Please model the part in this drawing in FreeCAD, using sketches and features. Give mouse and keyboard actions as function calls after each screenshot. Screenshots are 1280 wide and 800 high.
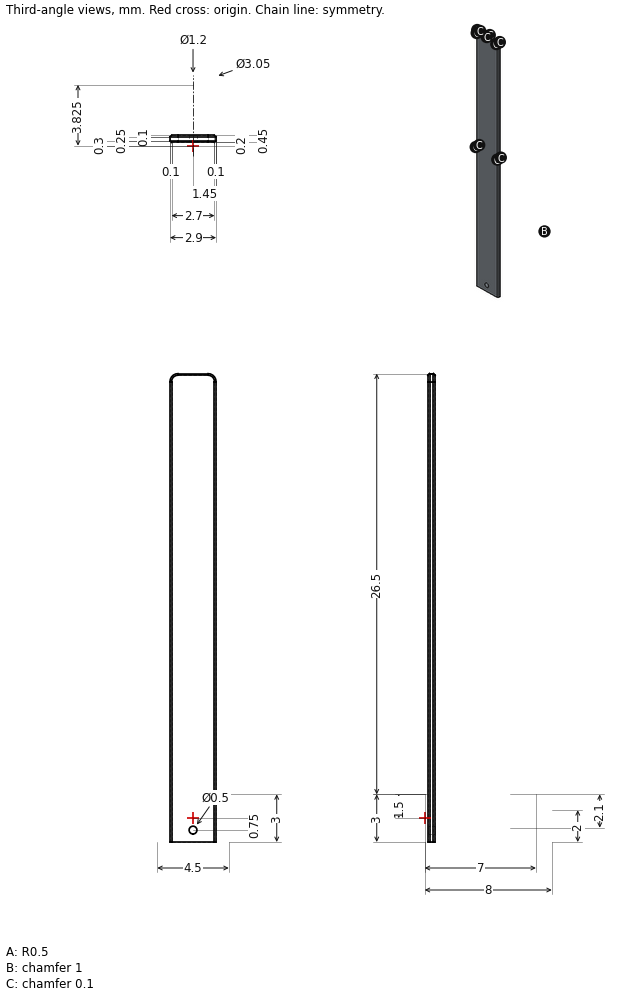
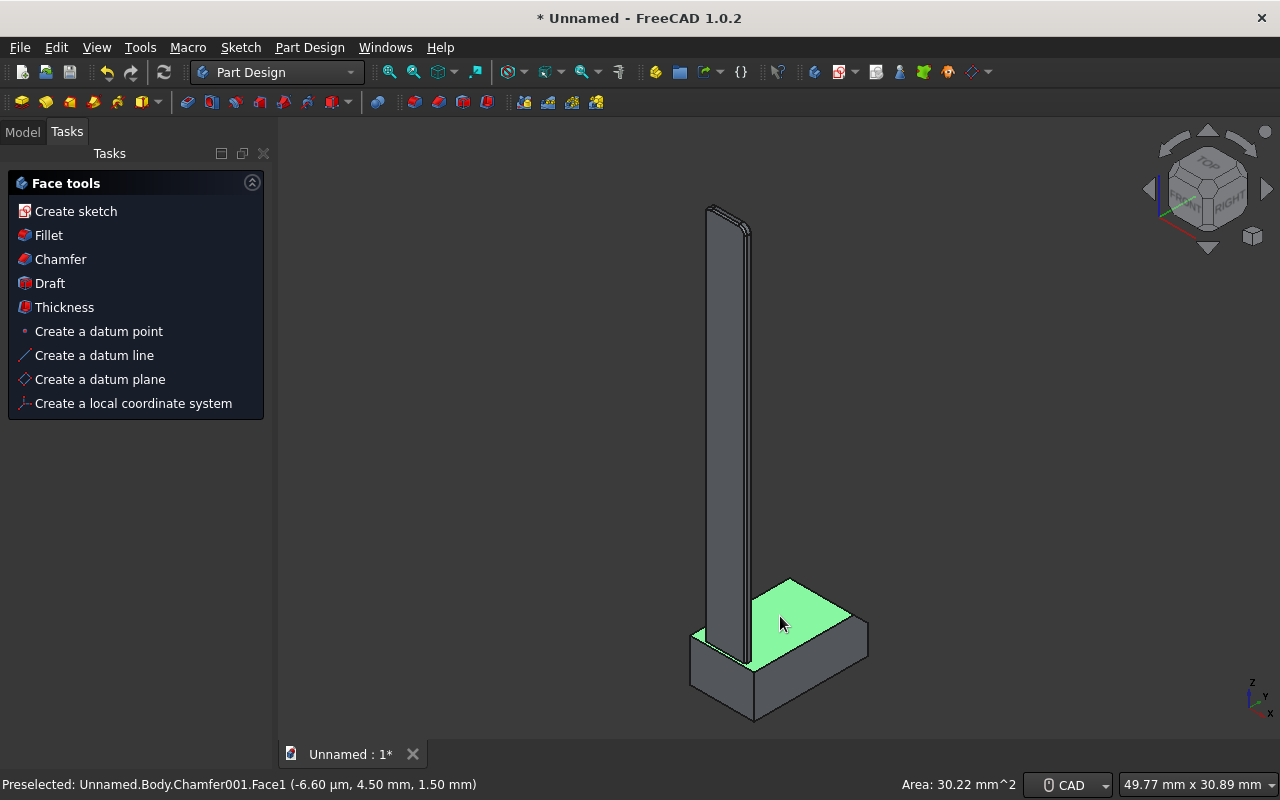
click(840, 72)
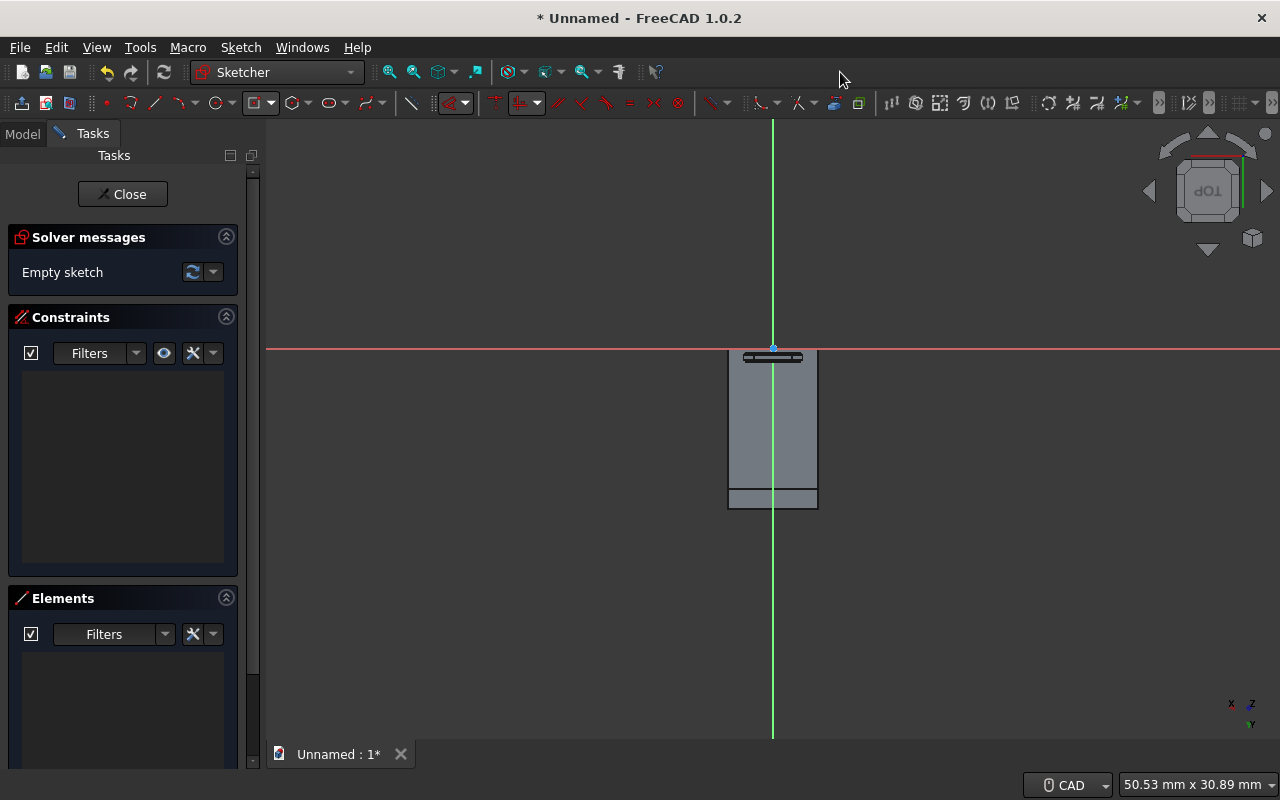
key(q)
key(s)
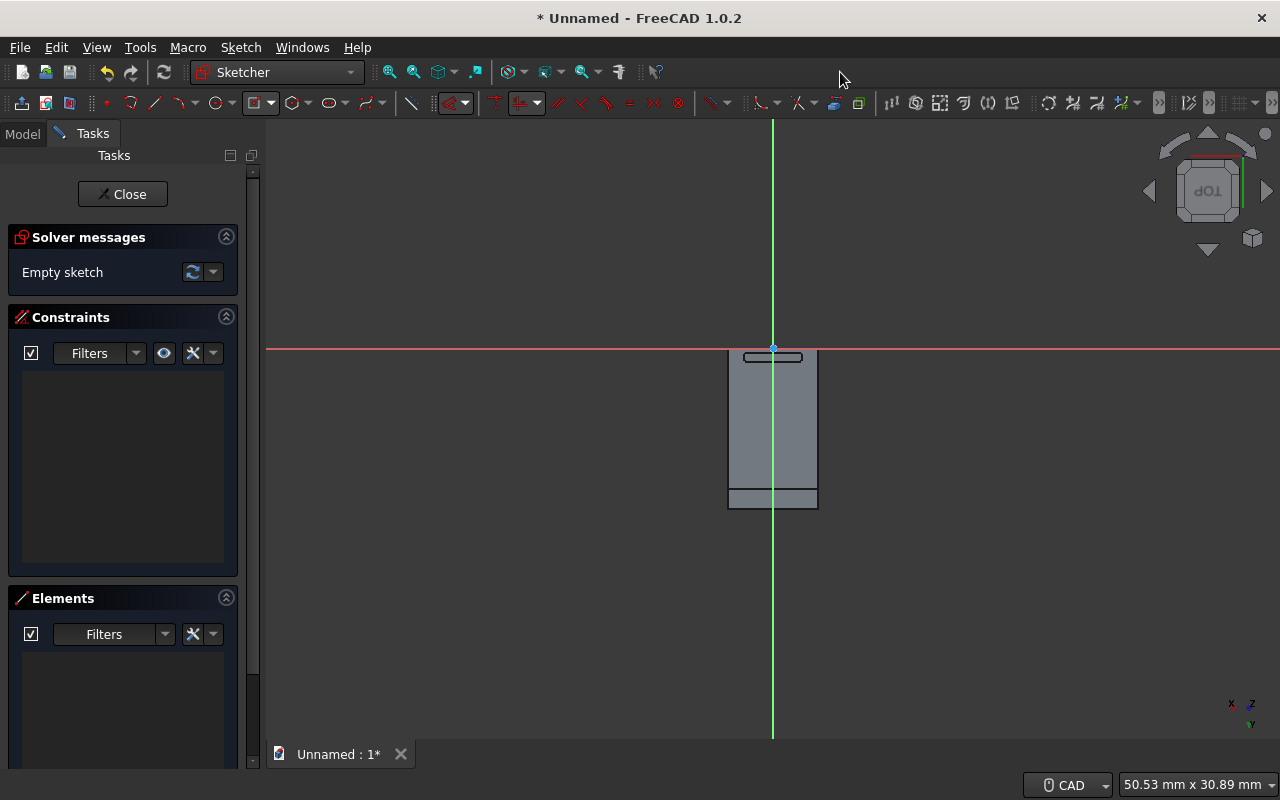
scroll(795, 394, up, 7)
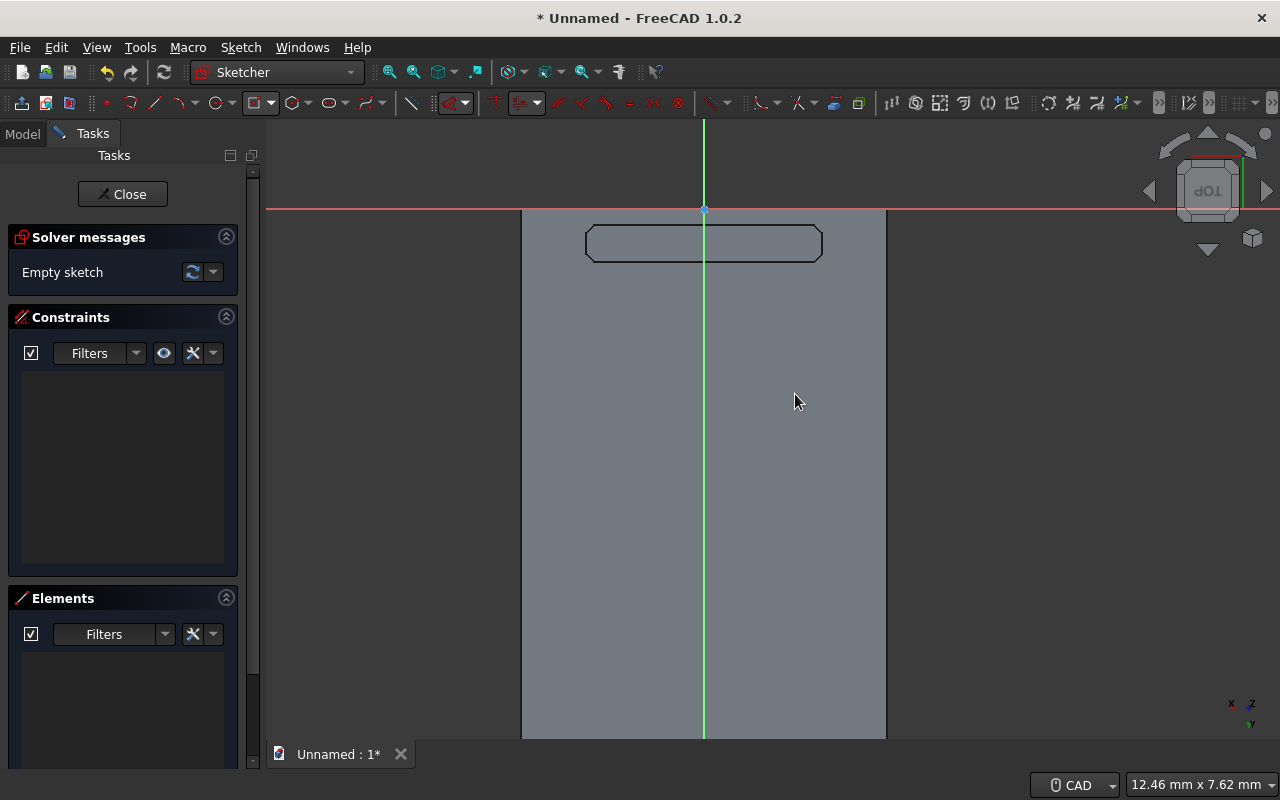
click(216, 104)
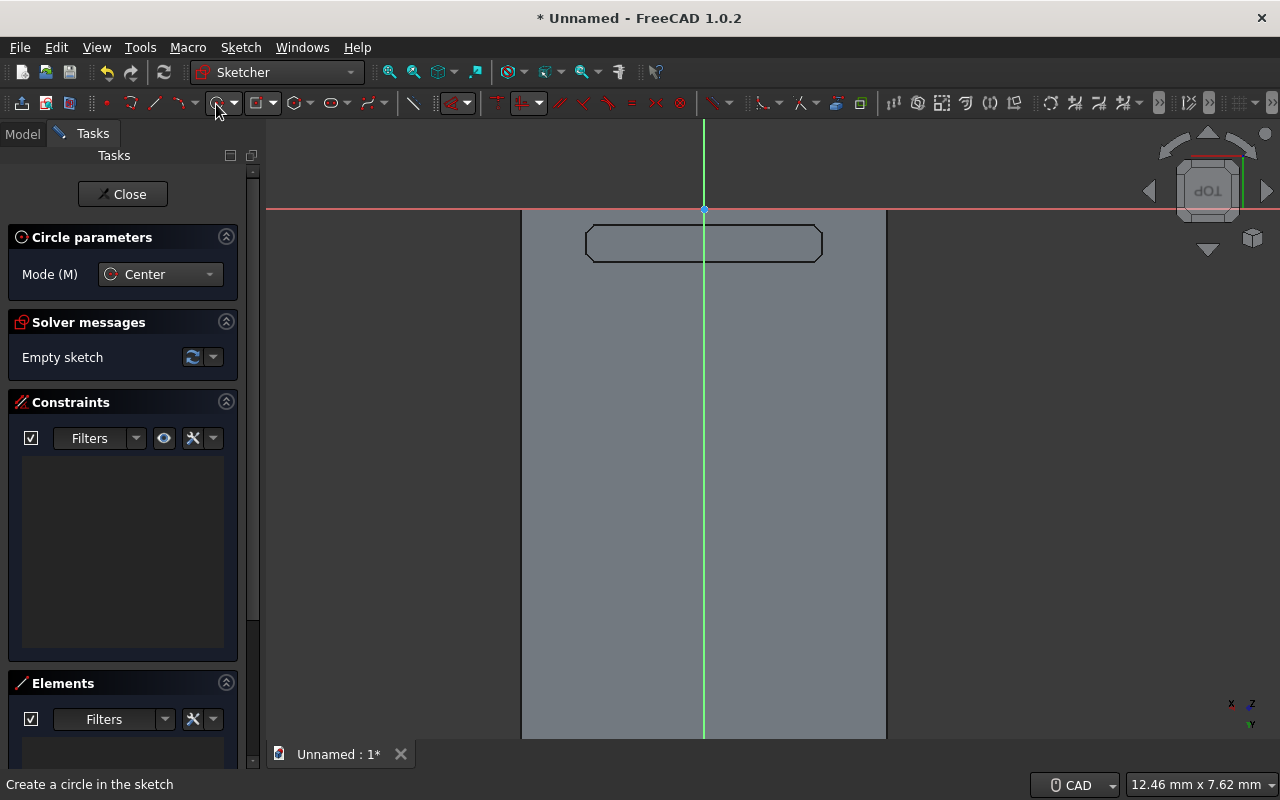
click(704, 520)
click(792, 433)
key(Escape)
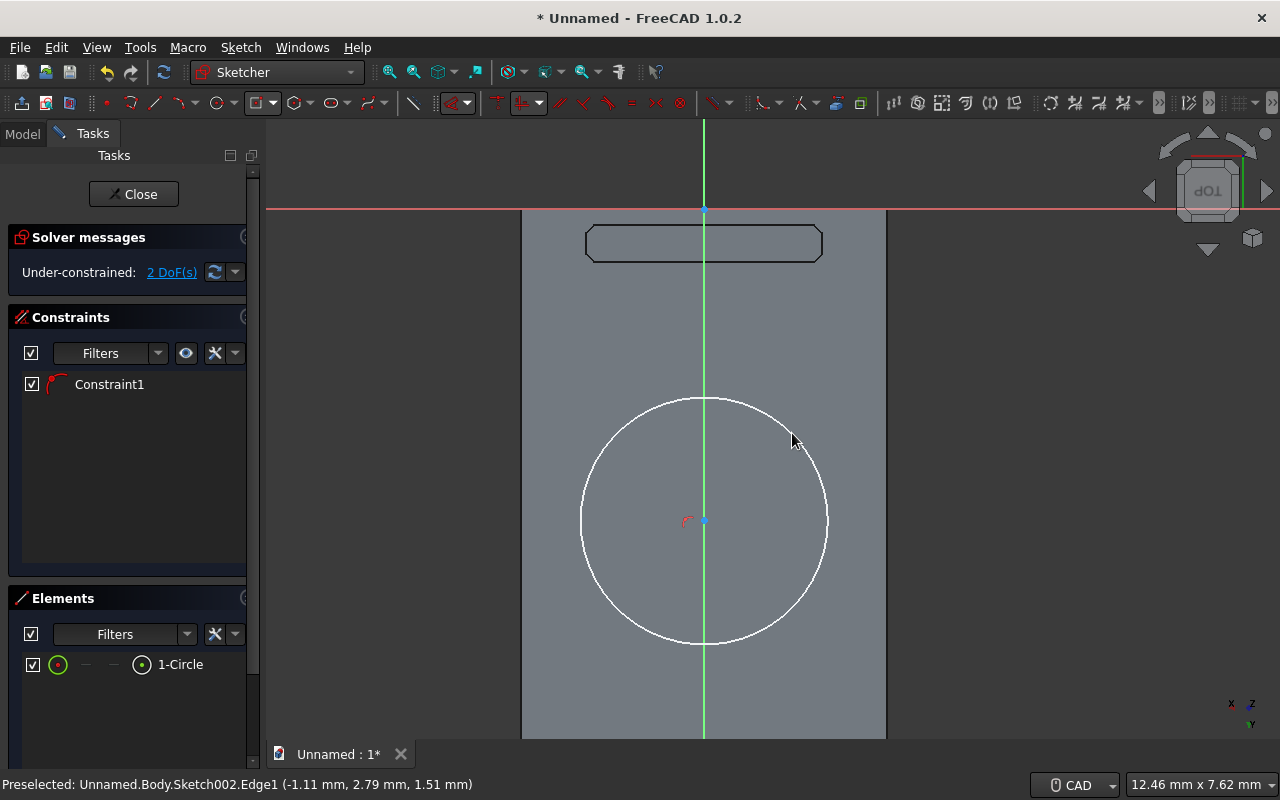
key(d)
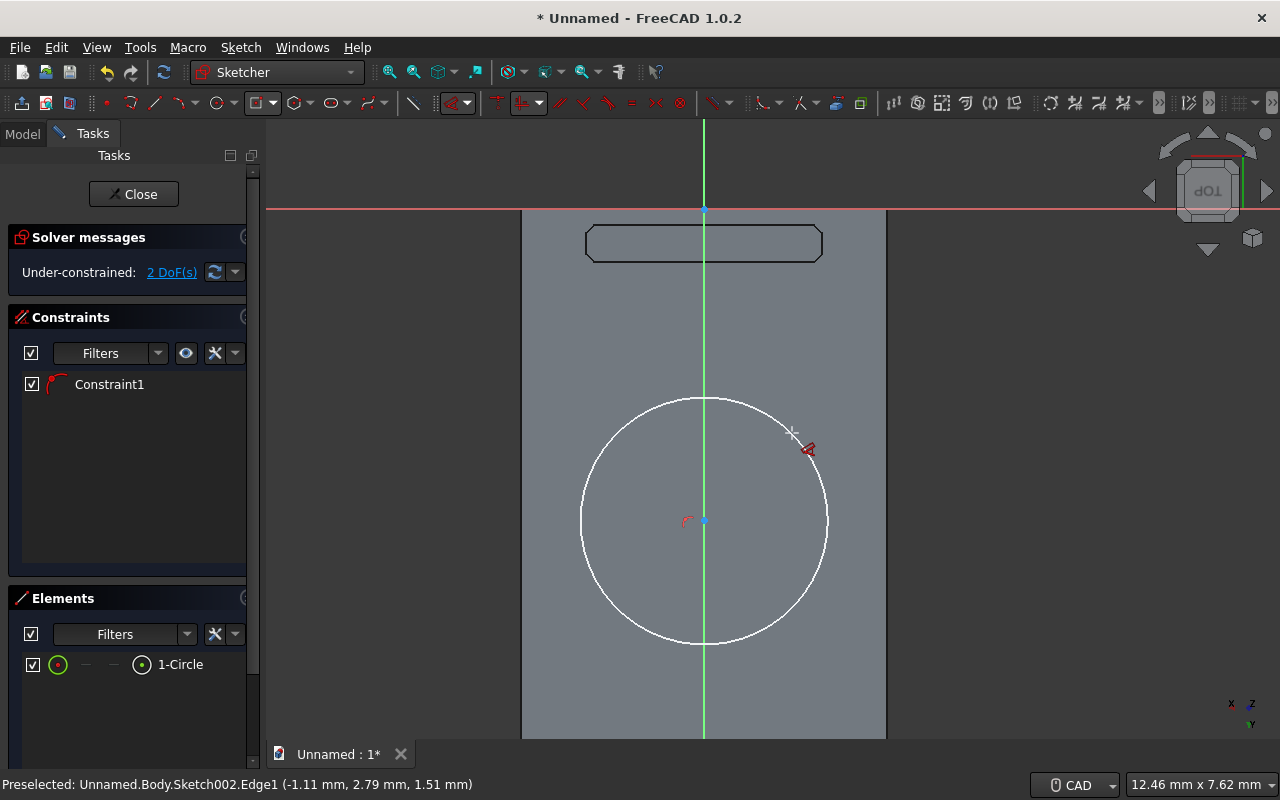
click(791, 433)
click(813, 410)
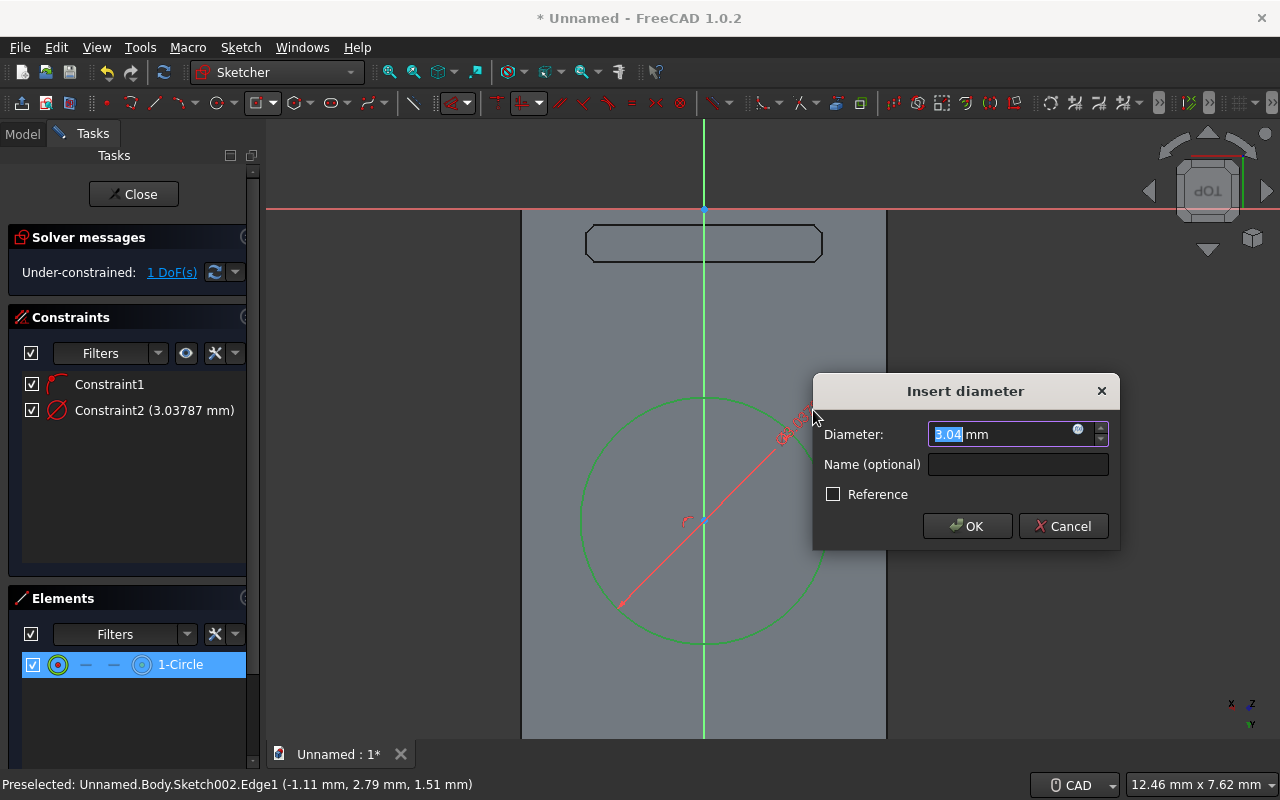
text(3.05)
key(Return)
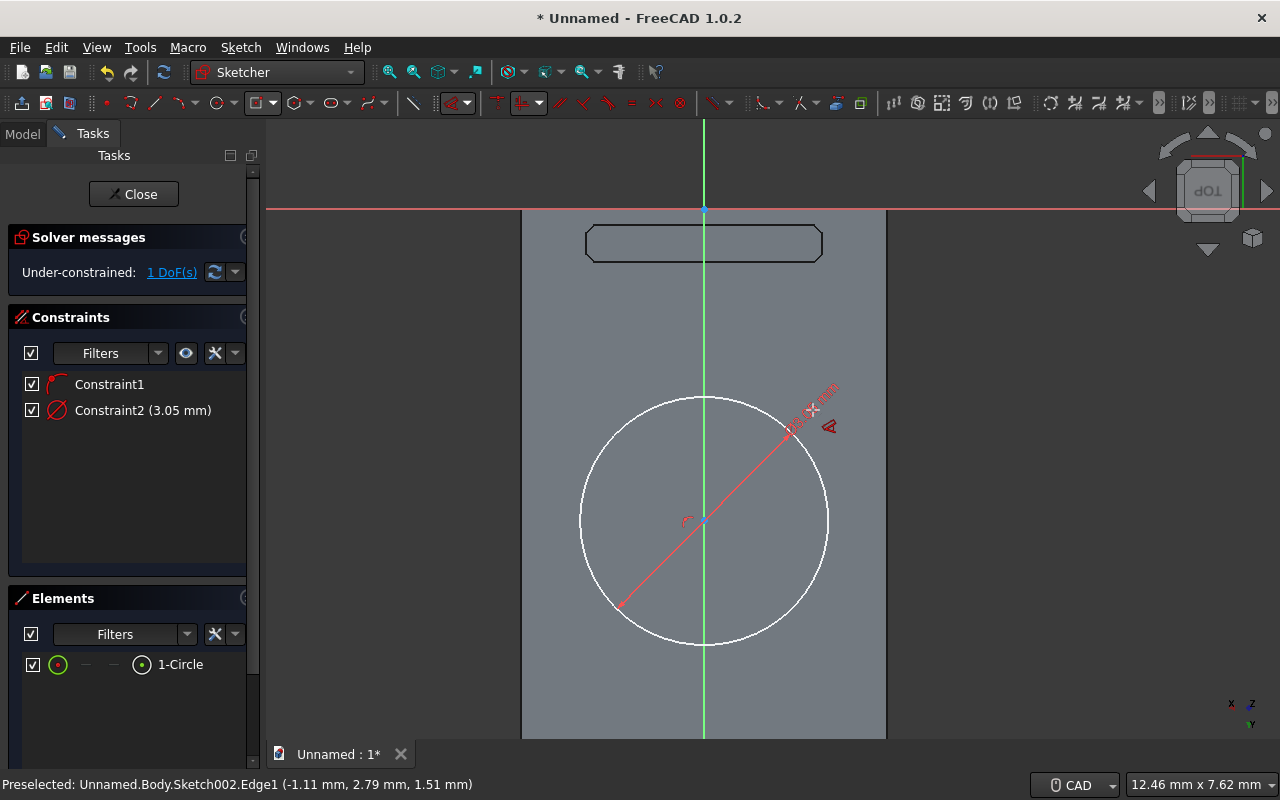
click(704, 521)
click(738, 365)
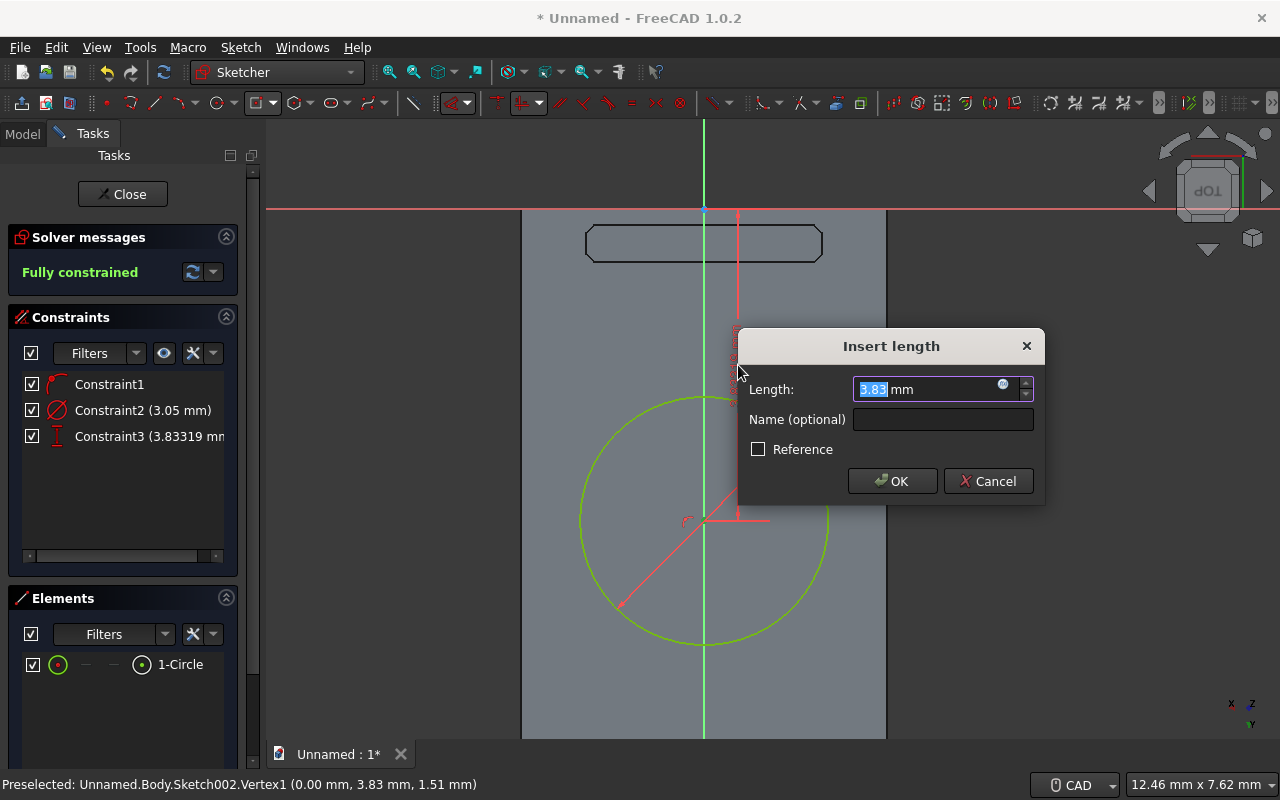
text(3.825)
key(Return)
key(Escape)